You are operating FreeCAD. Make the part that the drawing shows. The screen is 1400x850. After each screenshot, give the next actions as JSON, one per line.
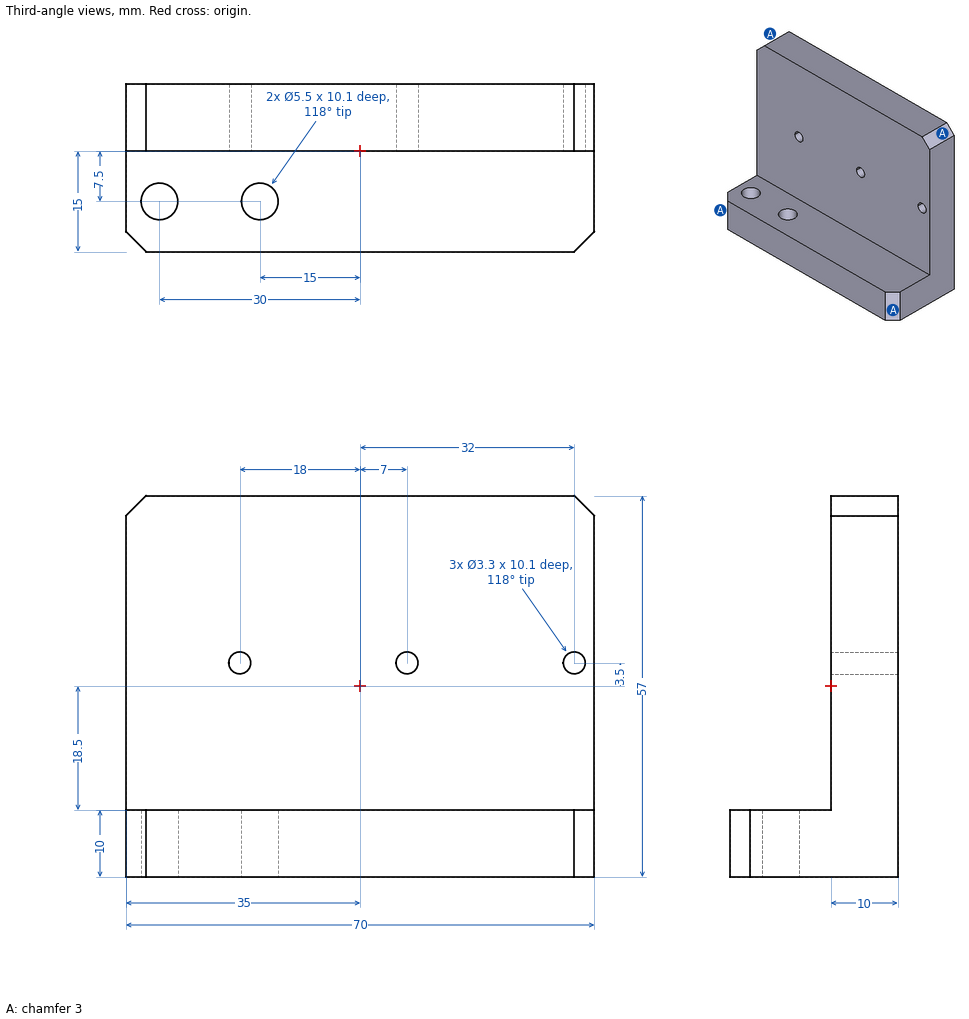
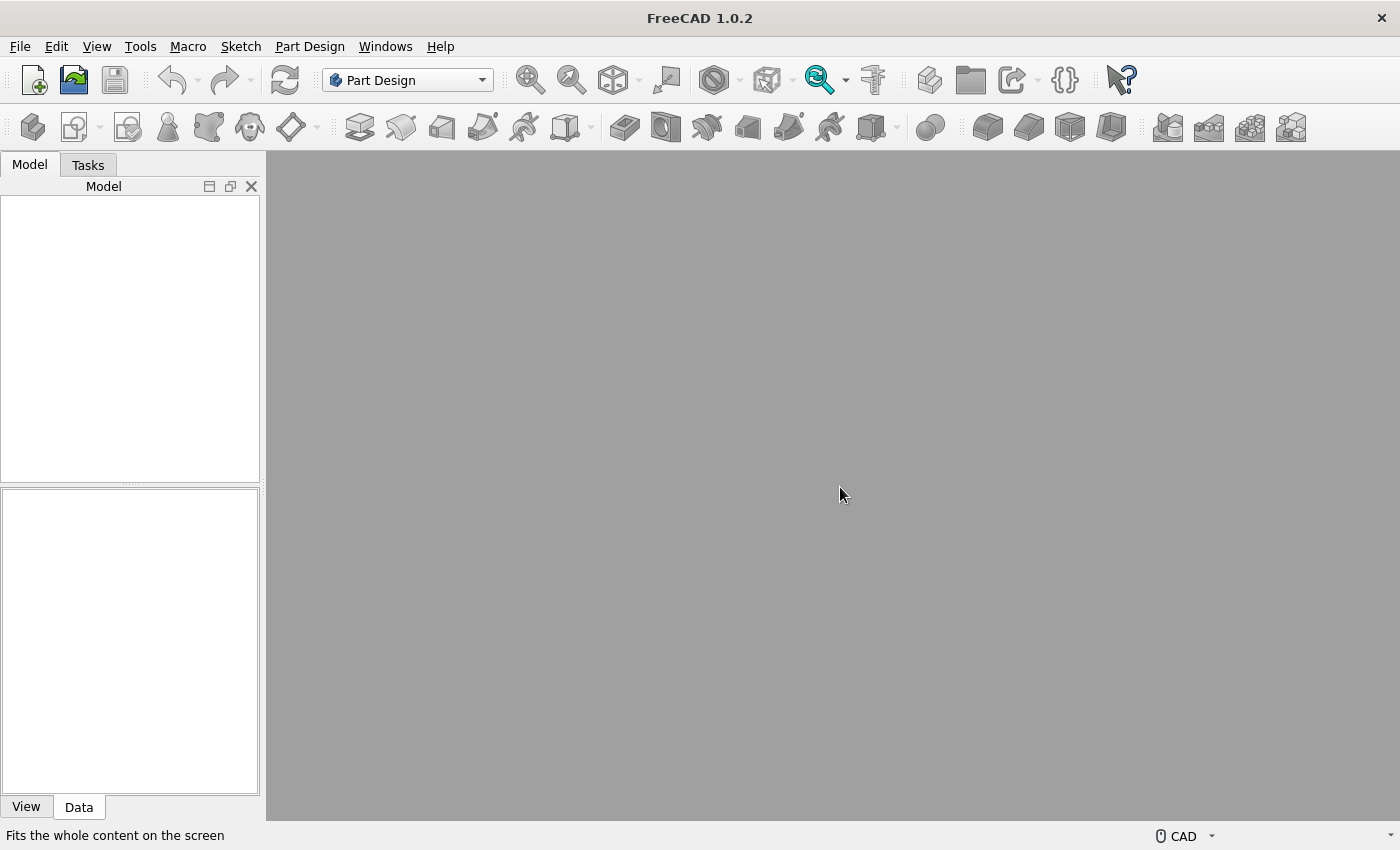
{"action": "left_click", "coordinate": [33, 80]}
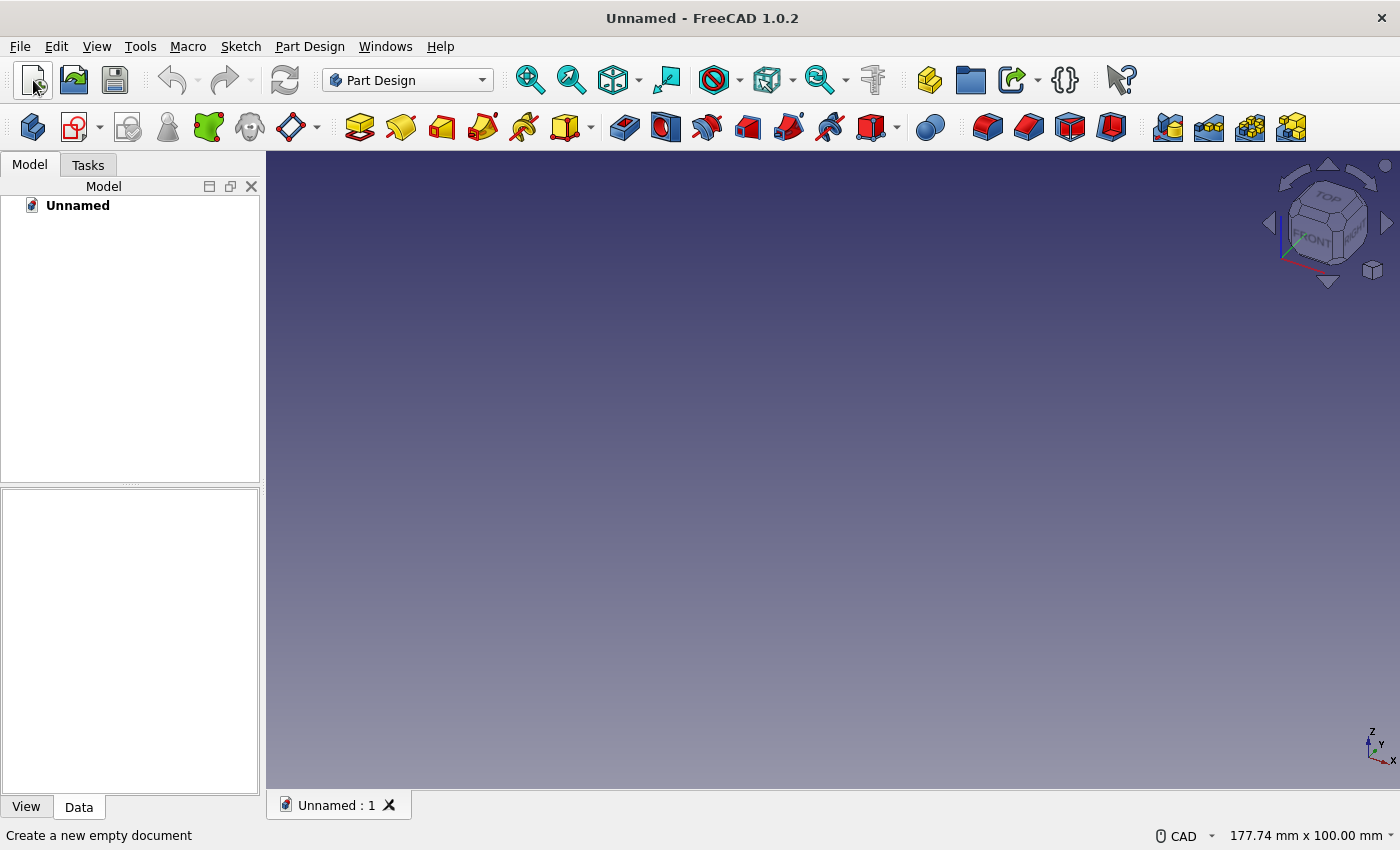
{"action": "left_click", "coordinate": [74, 128]}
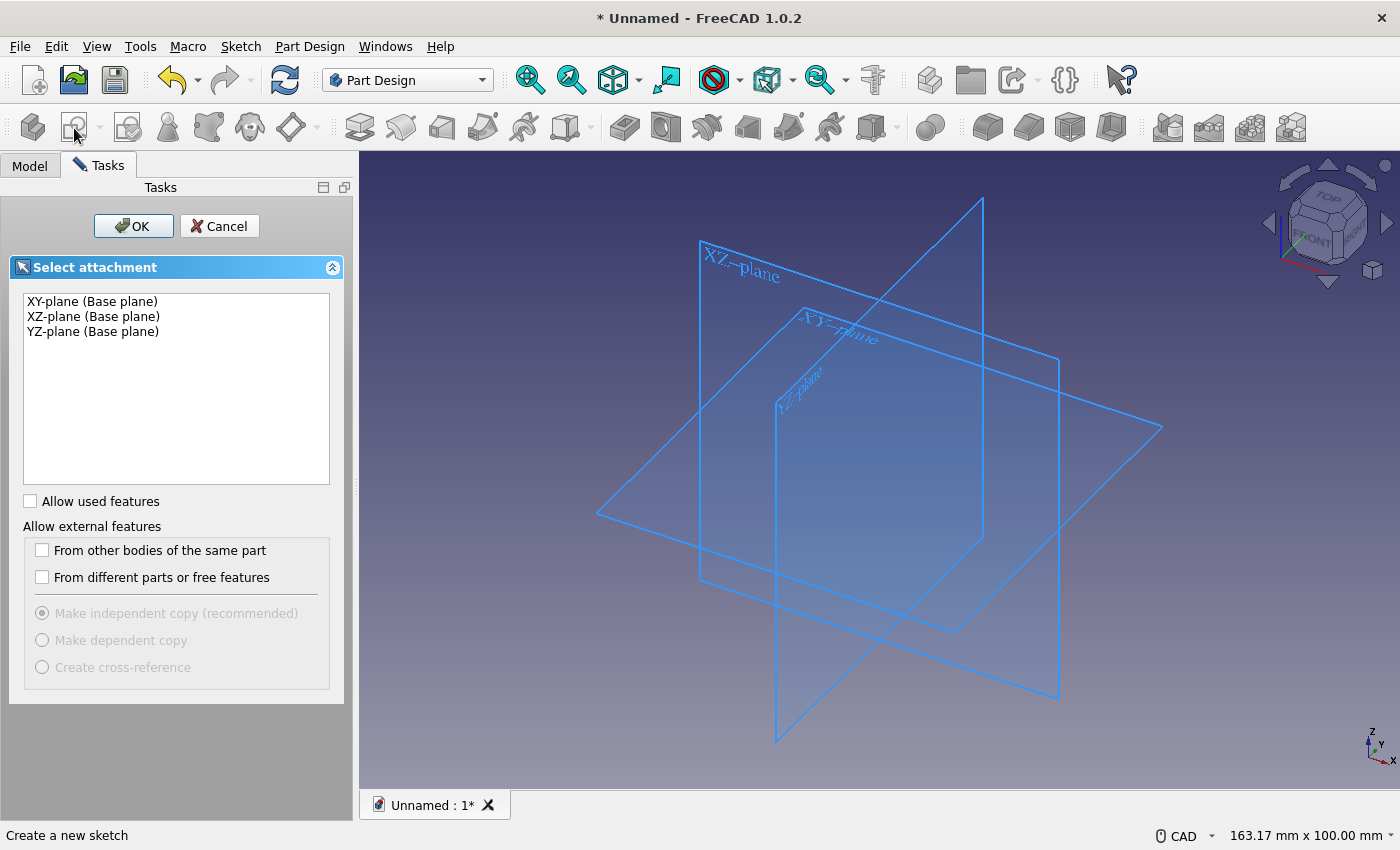
{"action": "left_click", "coordinate": [84, 316]}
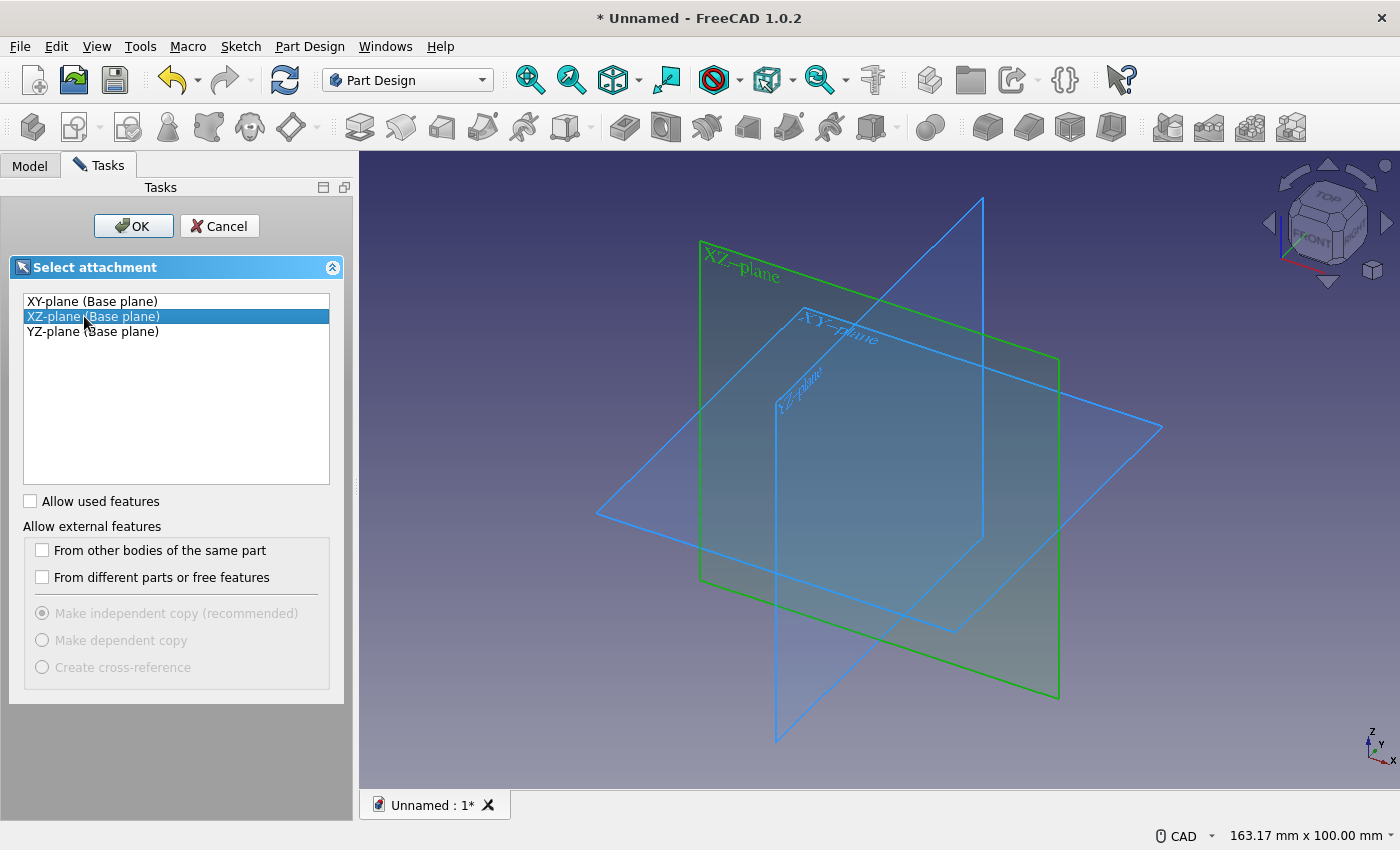
{"action": "left_click", "coordinate": [134, 226]}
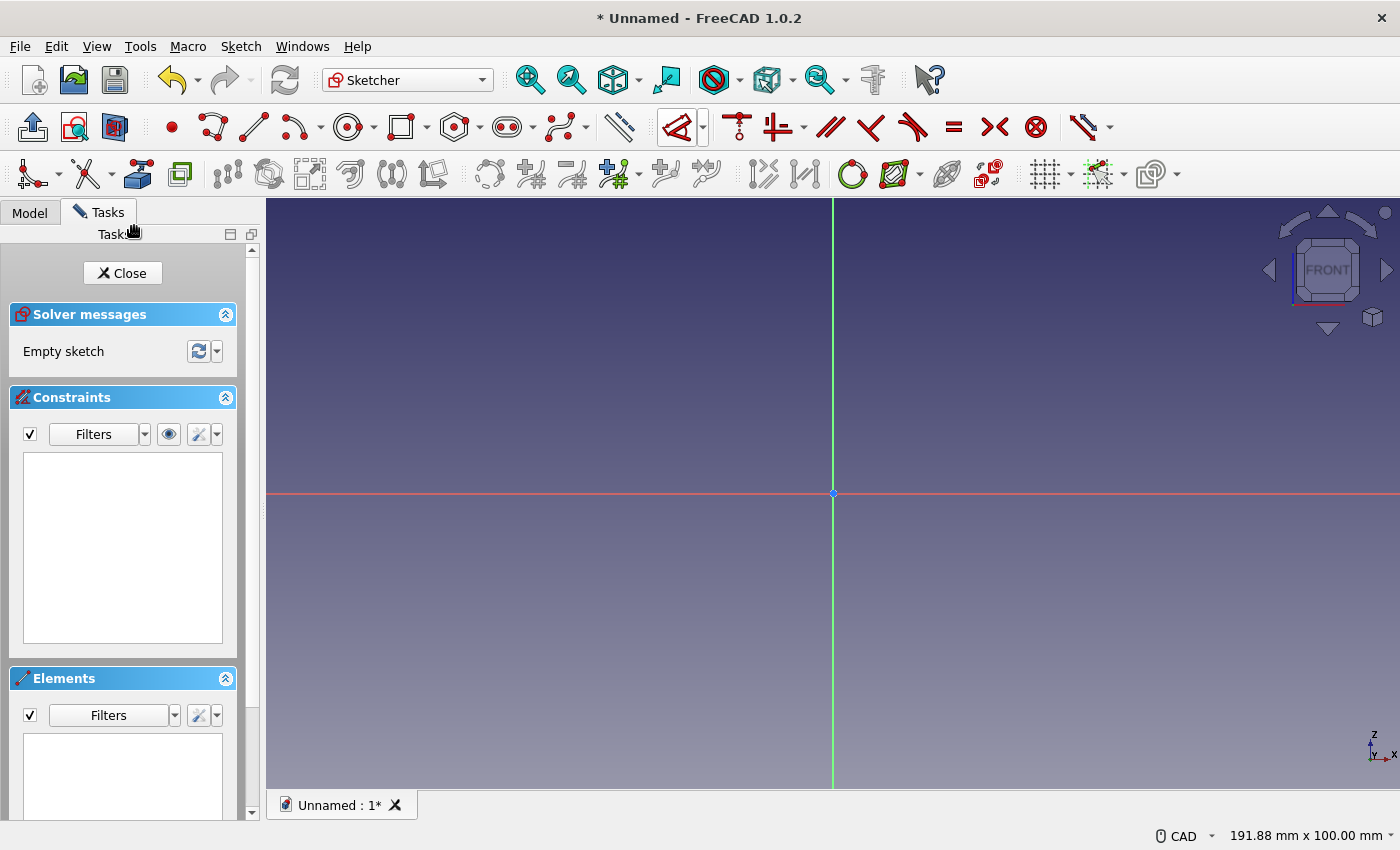
{"action": "key", "text": "g v"}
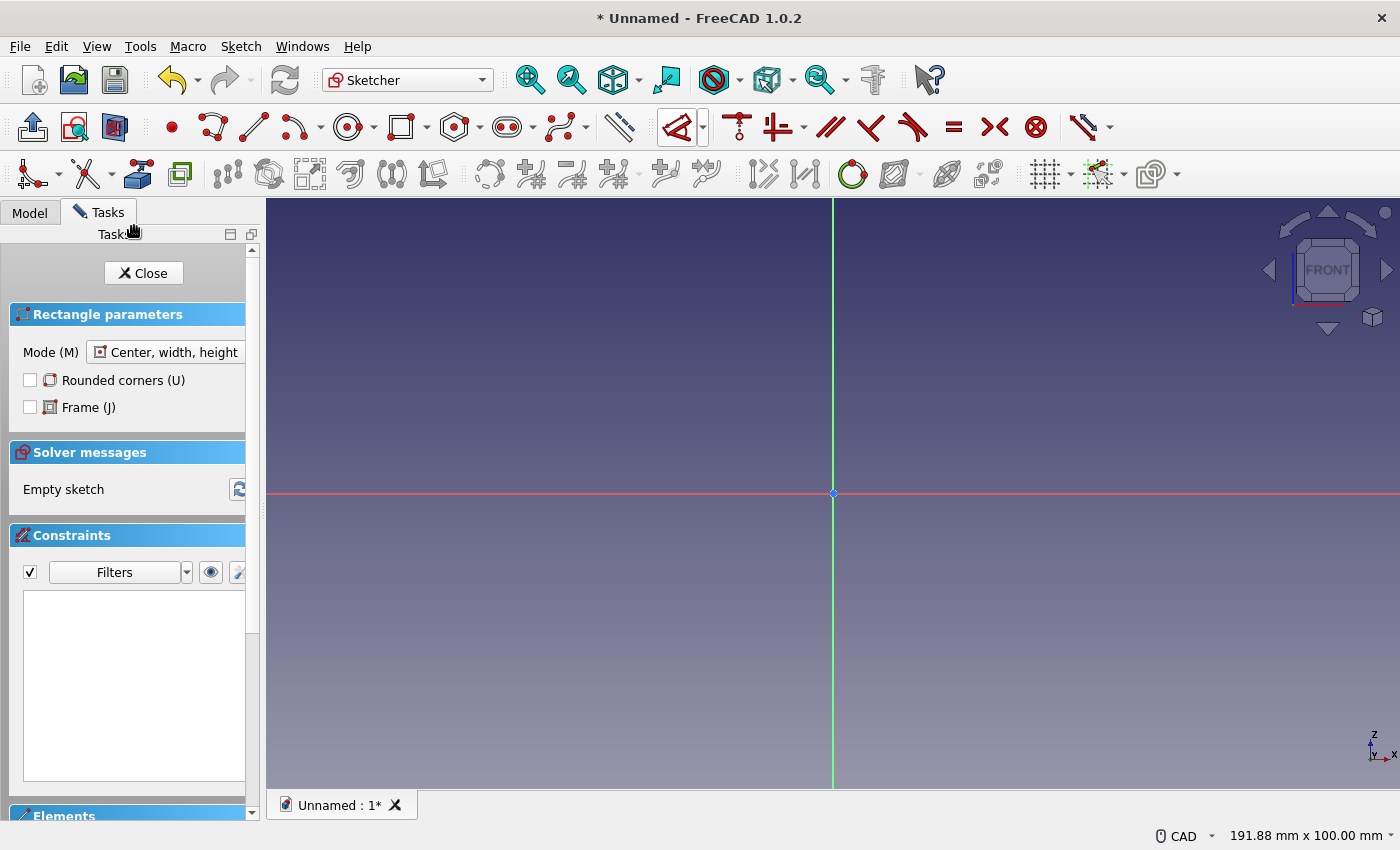
{"action": "left_click", "coordinate": [833, 494]}
{"action": "left_click", "coordinate": [1040, 325]}
{"action": "key", "text": "Escape"}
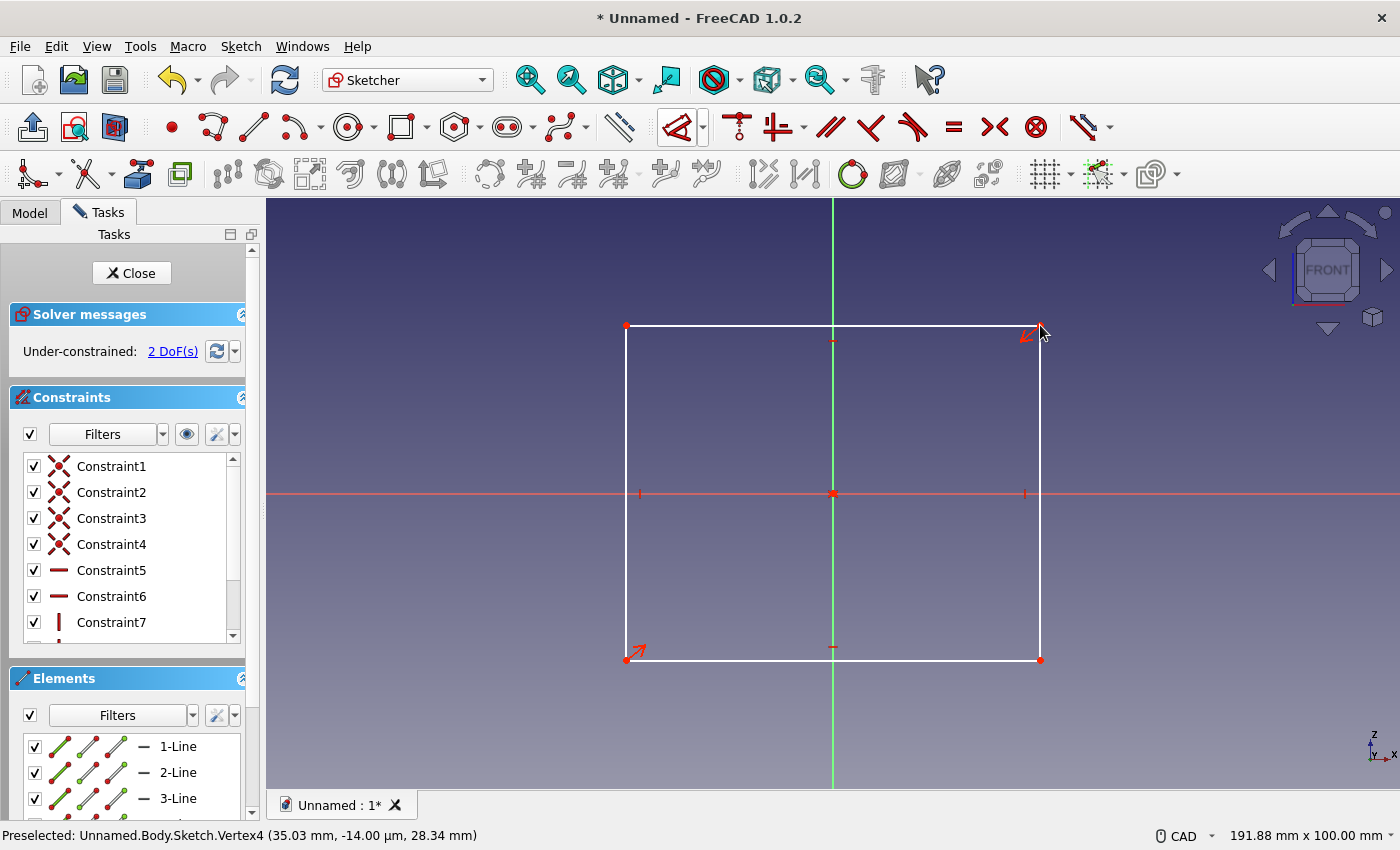
{"action": "left_click", "coordinate": [676, 128]}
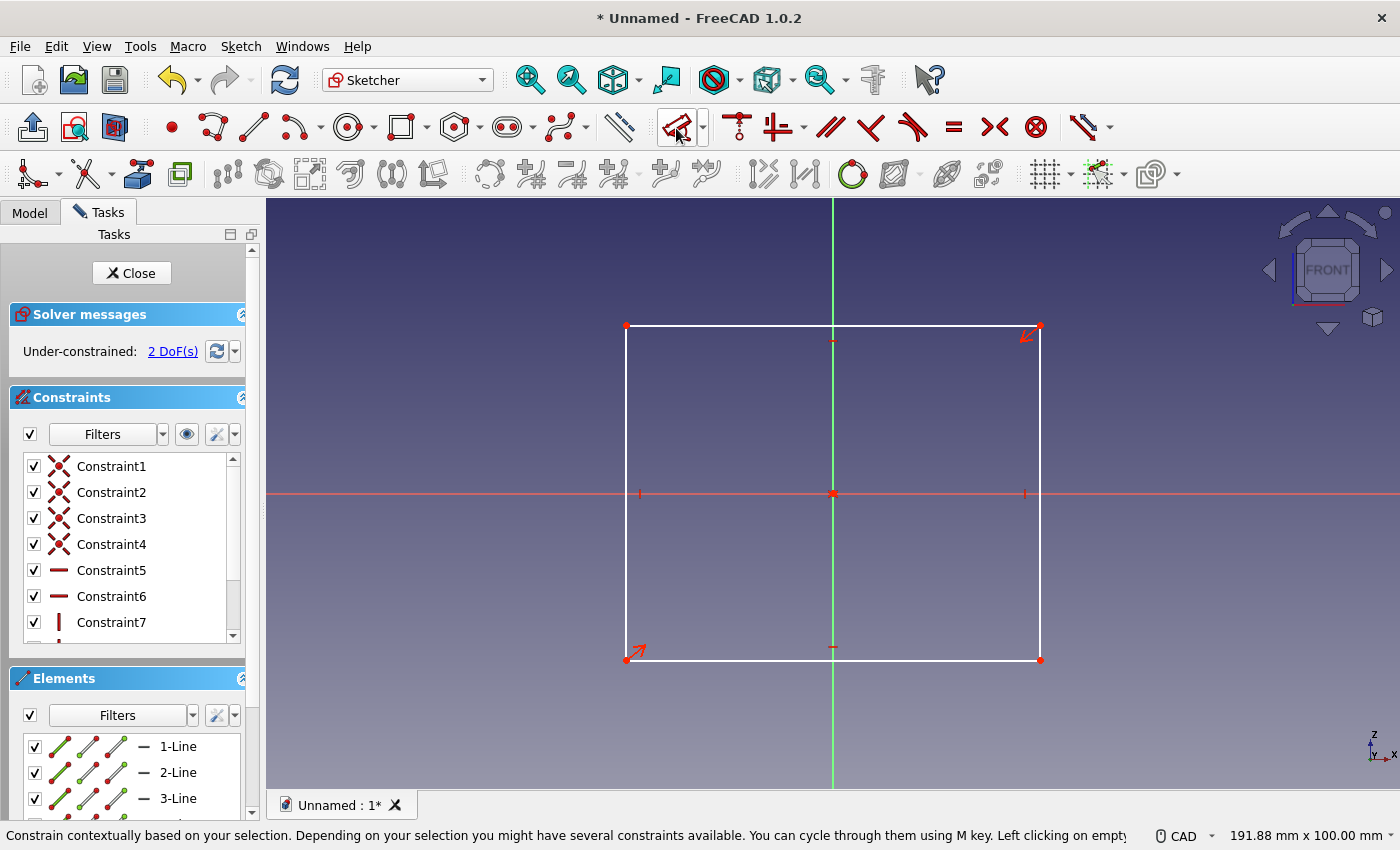
{"action": "left_click", "coordinate": [750, 661]}
{"action": "left_click", "coordinate": [738, 695]}